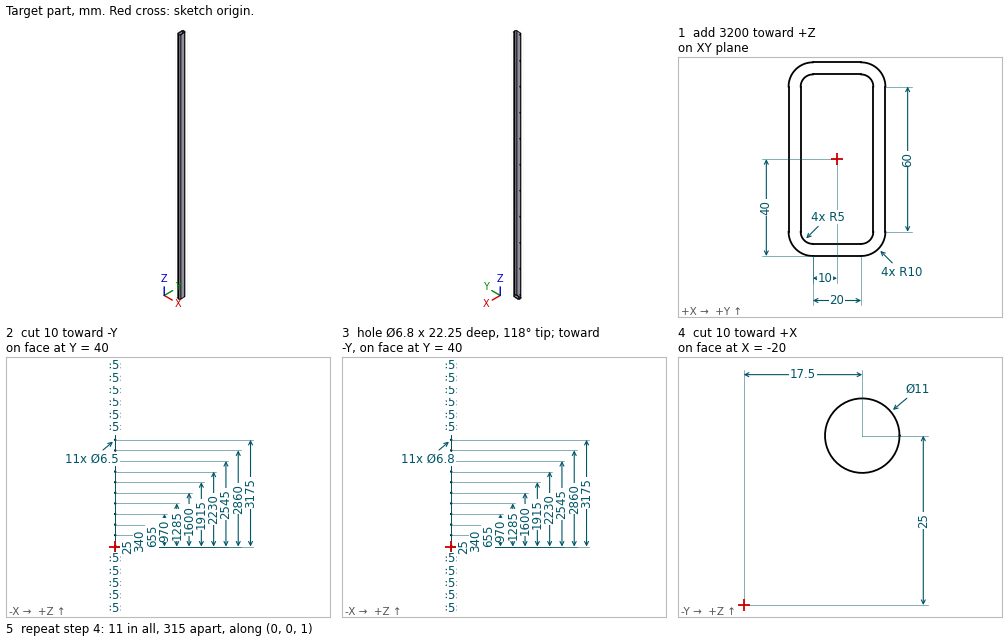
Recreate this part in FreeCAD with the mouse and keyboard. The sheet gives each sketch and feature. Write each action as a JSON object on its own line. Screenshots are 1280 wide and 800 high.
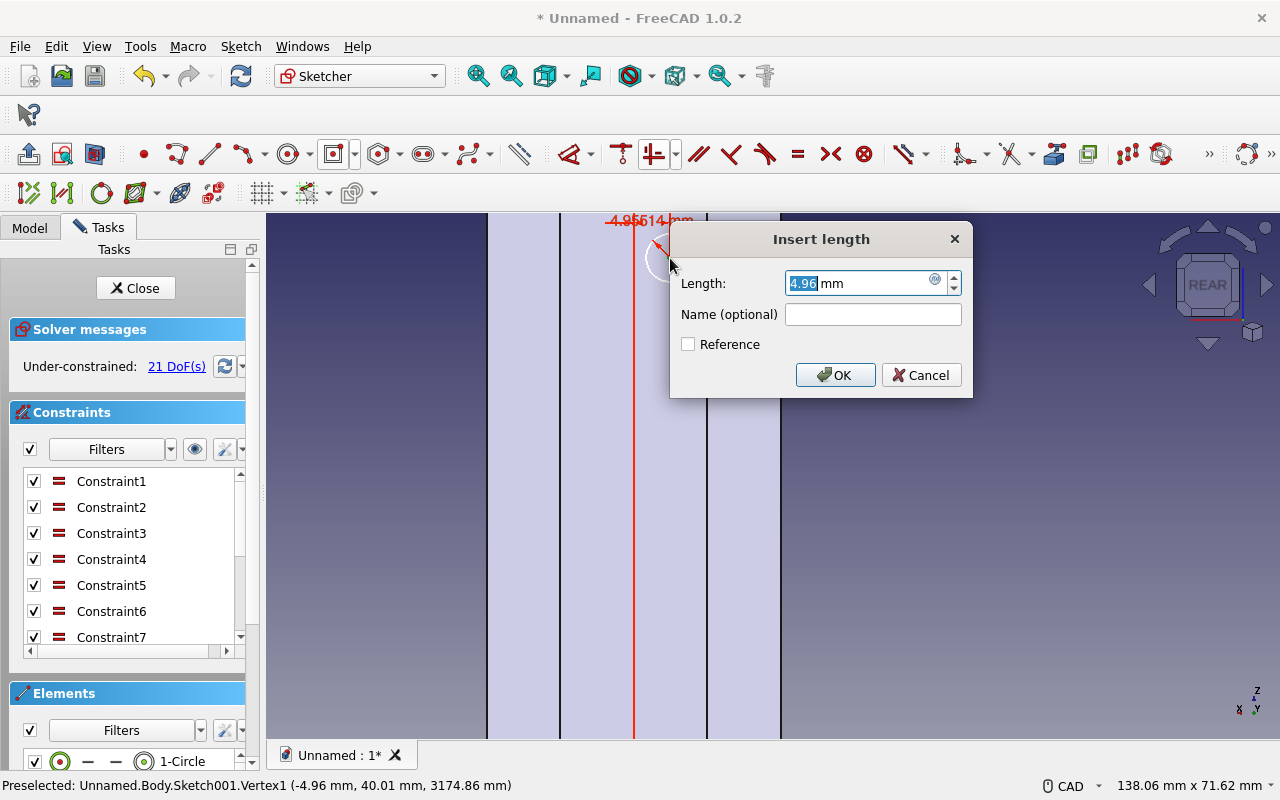
{"action": "type", "text": "5"}
{"action": "key", "text": "Return"}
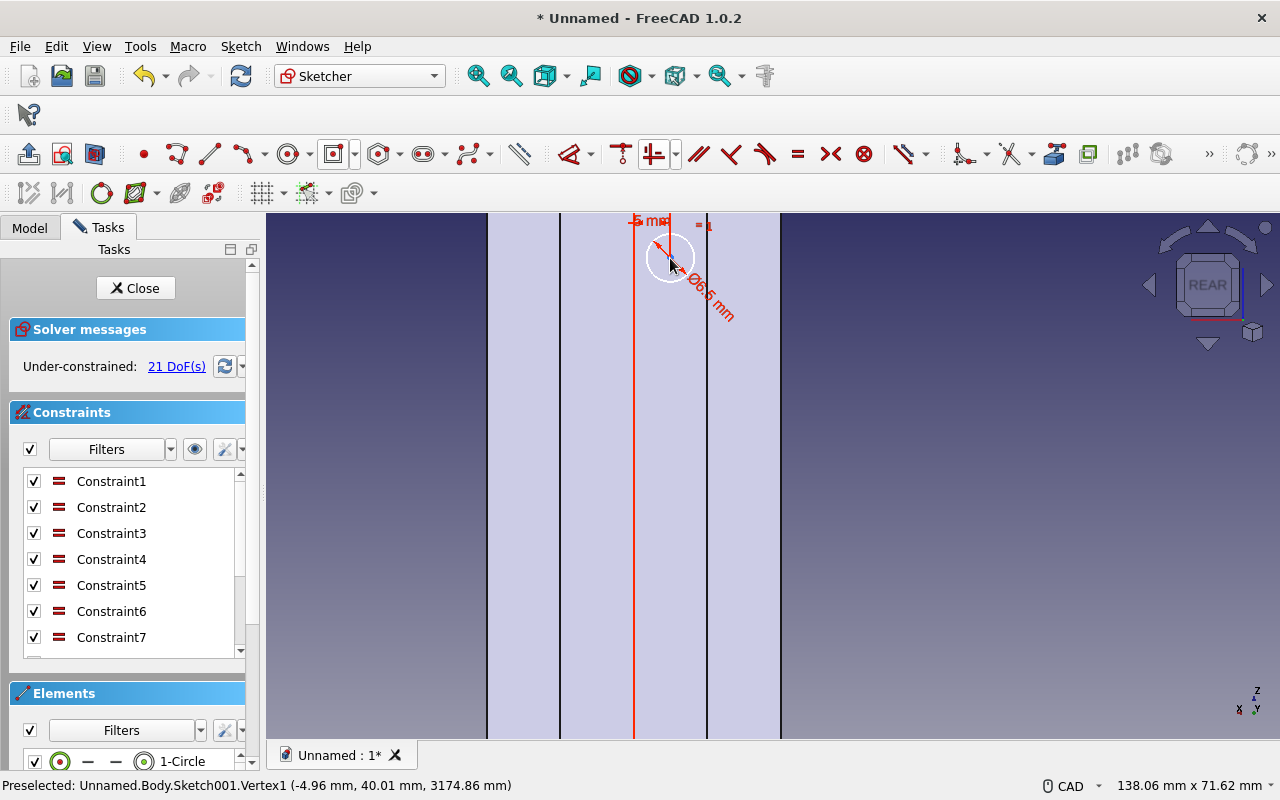
{"action": "scroll", "coordinate": [704, 476], "scroll_direction": "down", "scroll_amount": 15}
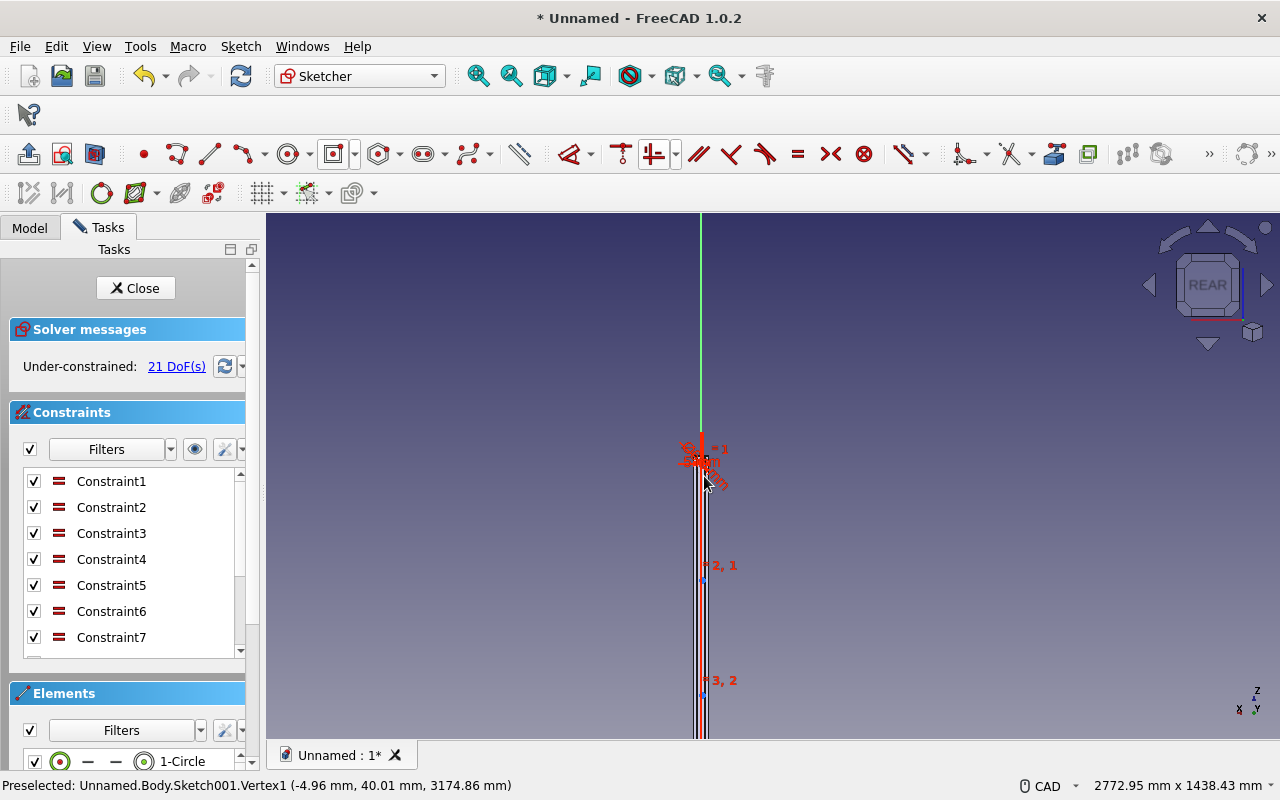
{"action": "scroll", "coordinate": [705, 241], "scroll_direction": "down", "scroll_amount": 6}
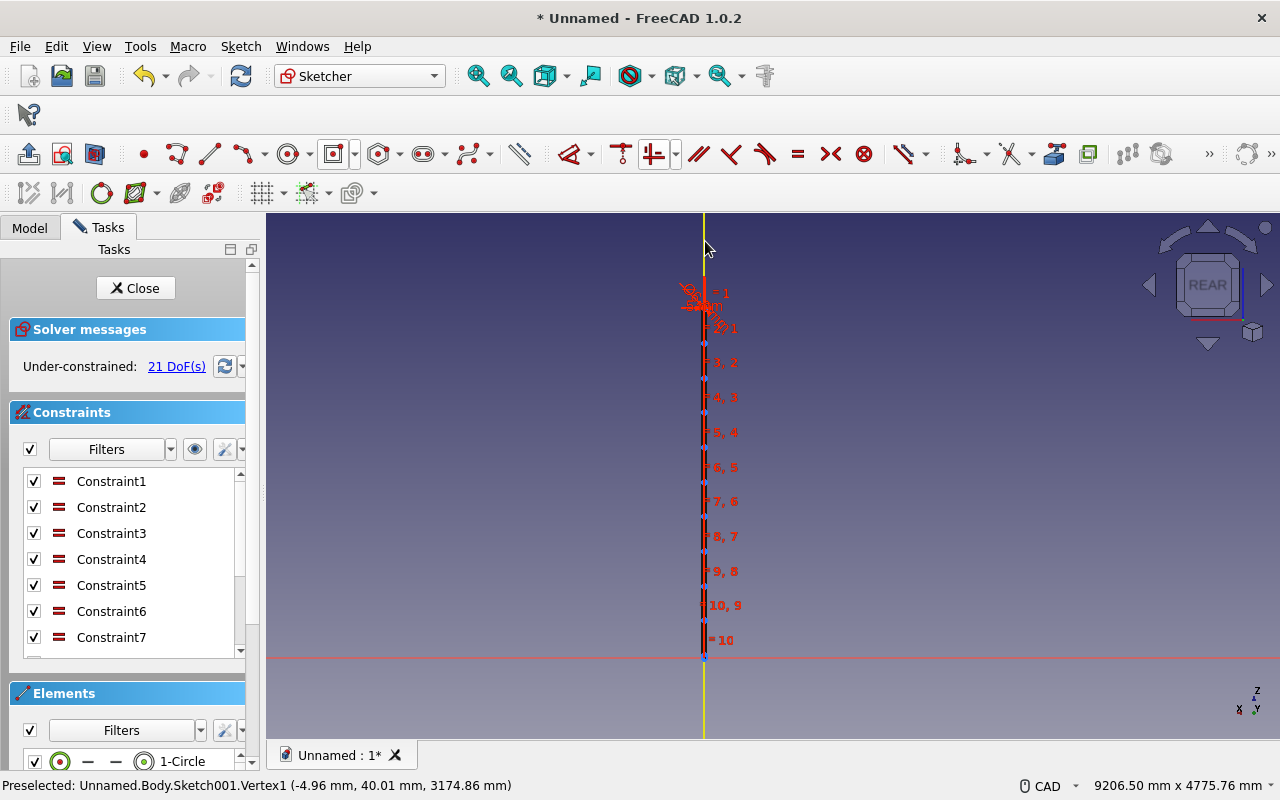
{"action": "scroll", "coordinate": [705, 343], "scroll_direction": "up", "scroll_amount": 22}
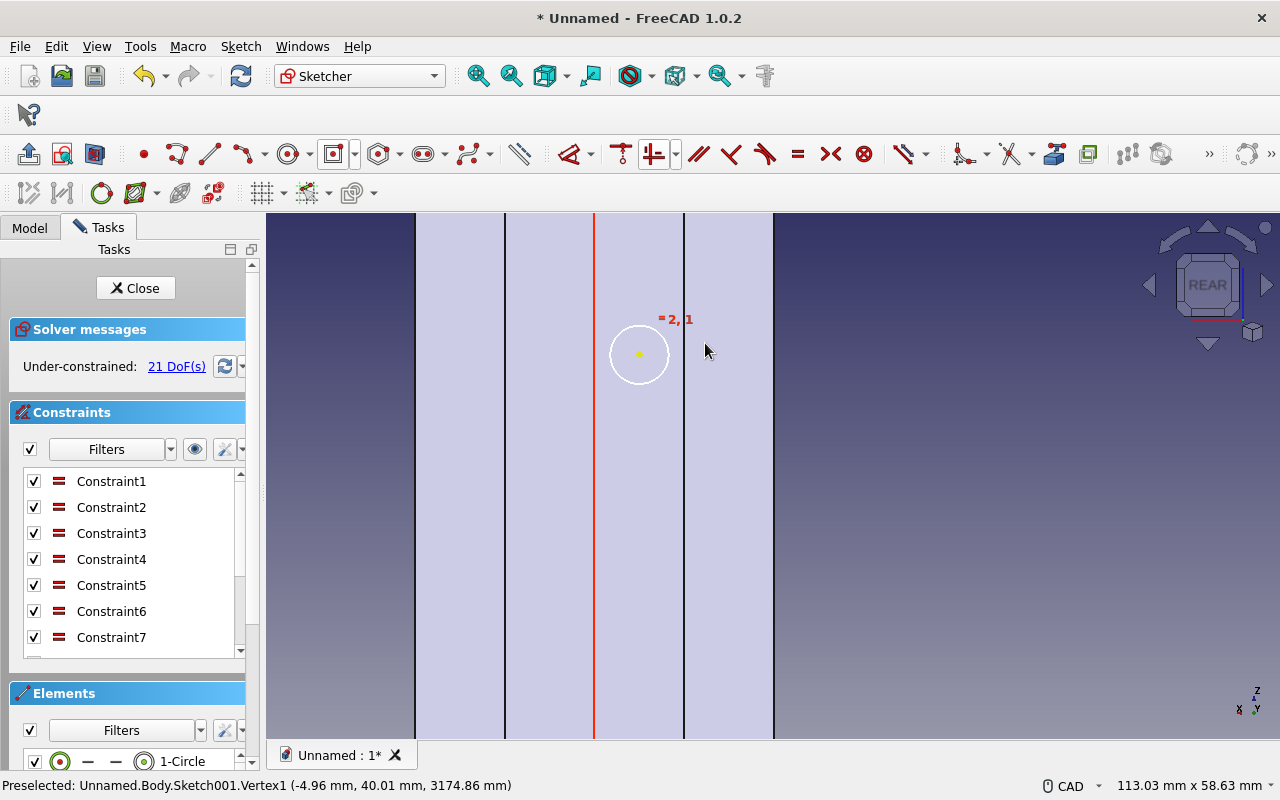
{"action": "left_click", "coordinate": [639, 355]}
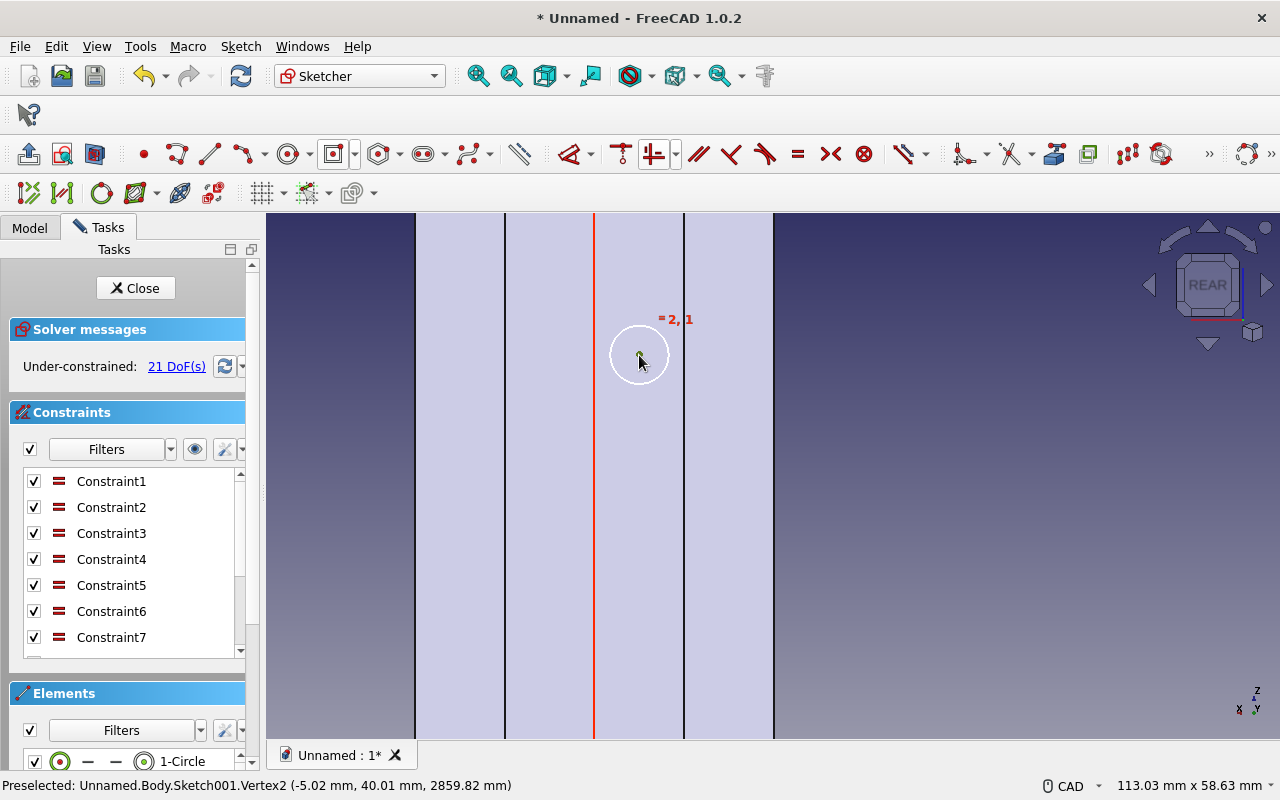
{"action": "key", "text": "l"}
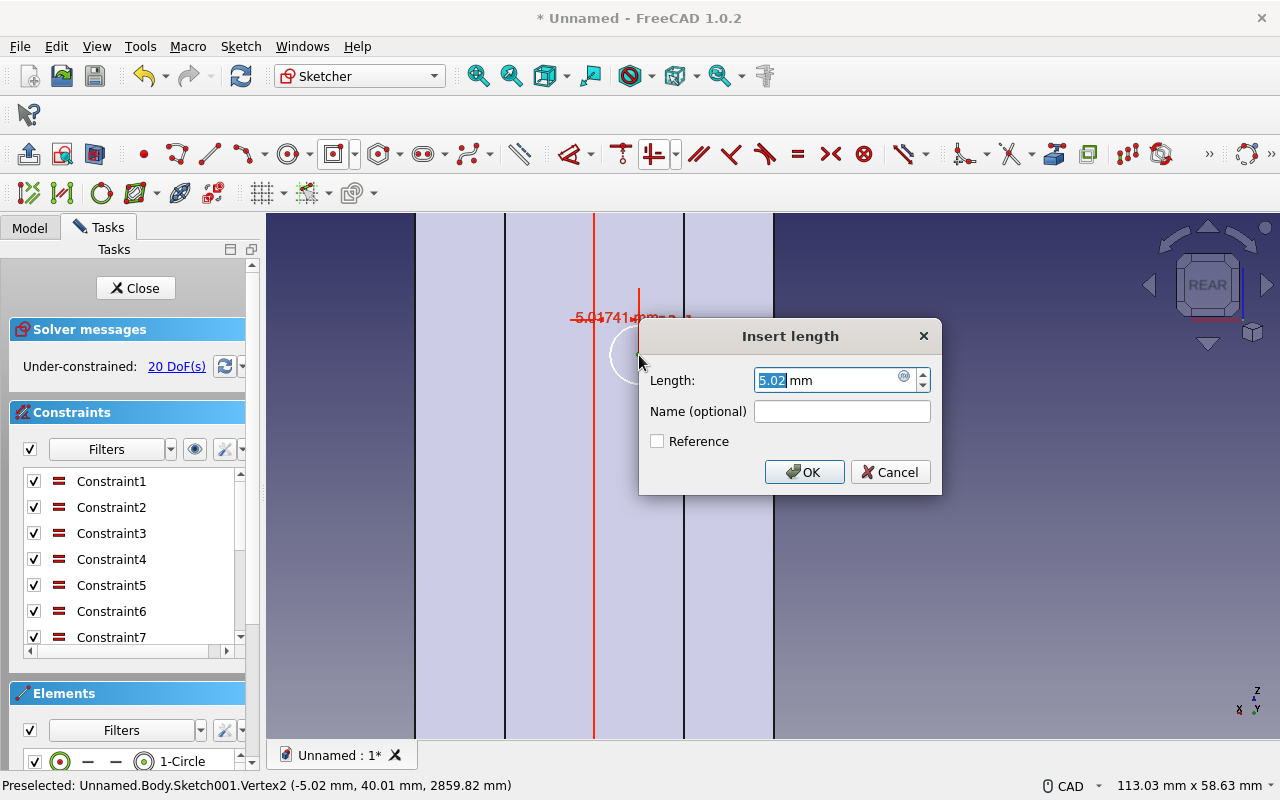
{"action": "type", "text": "5"}
{"action": "key", "text": "Return"}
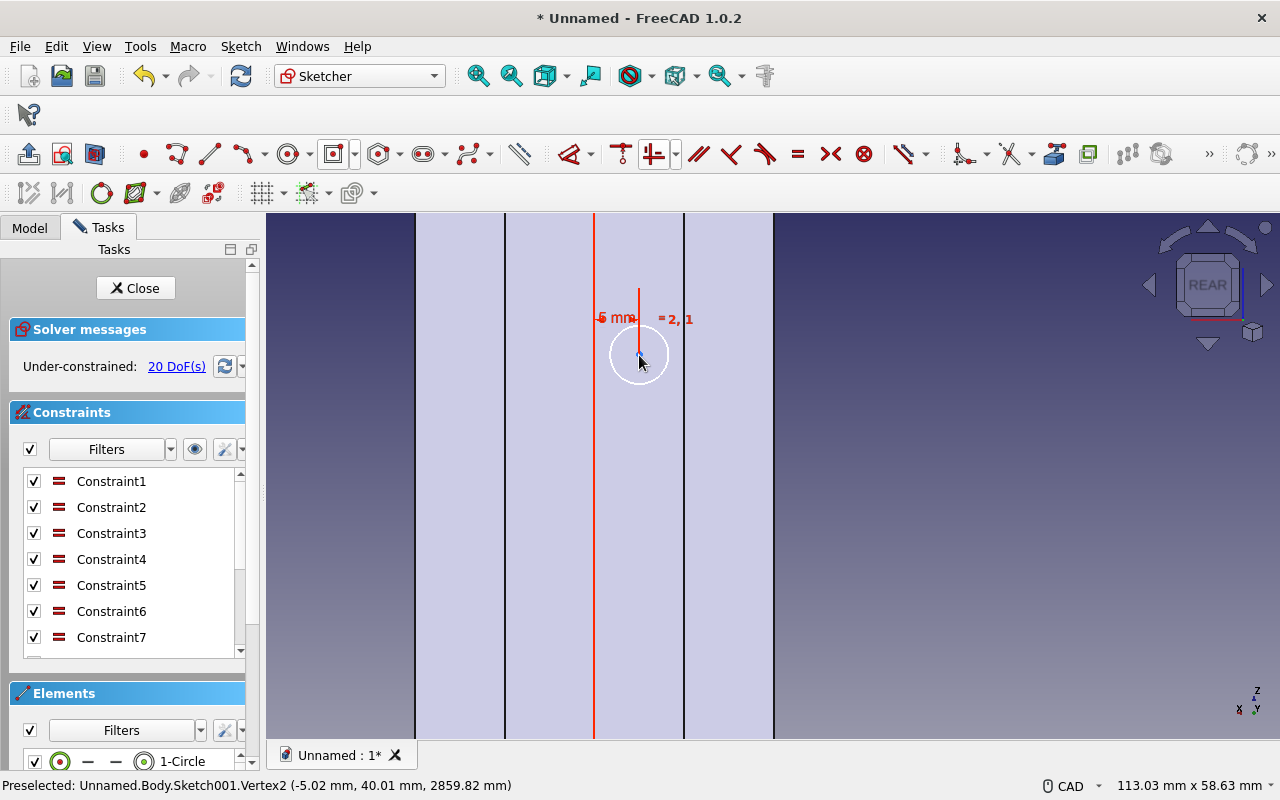
{"action": "scroll", "coordinate": [704, 476], "scroll_direction": "down", "scroll_amount": 15}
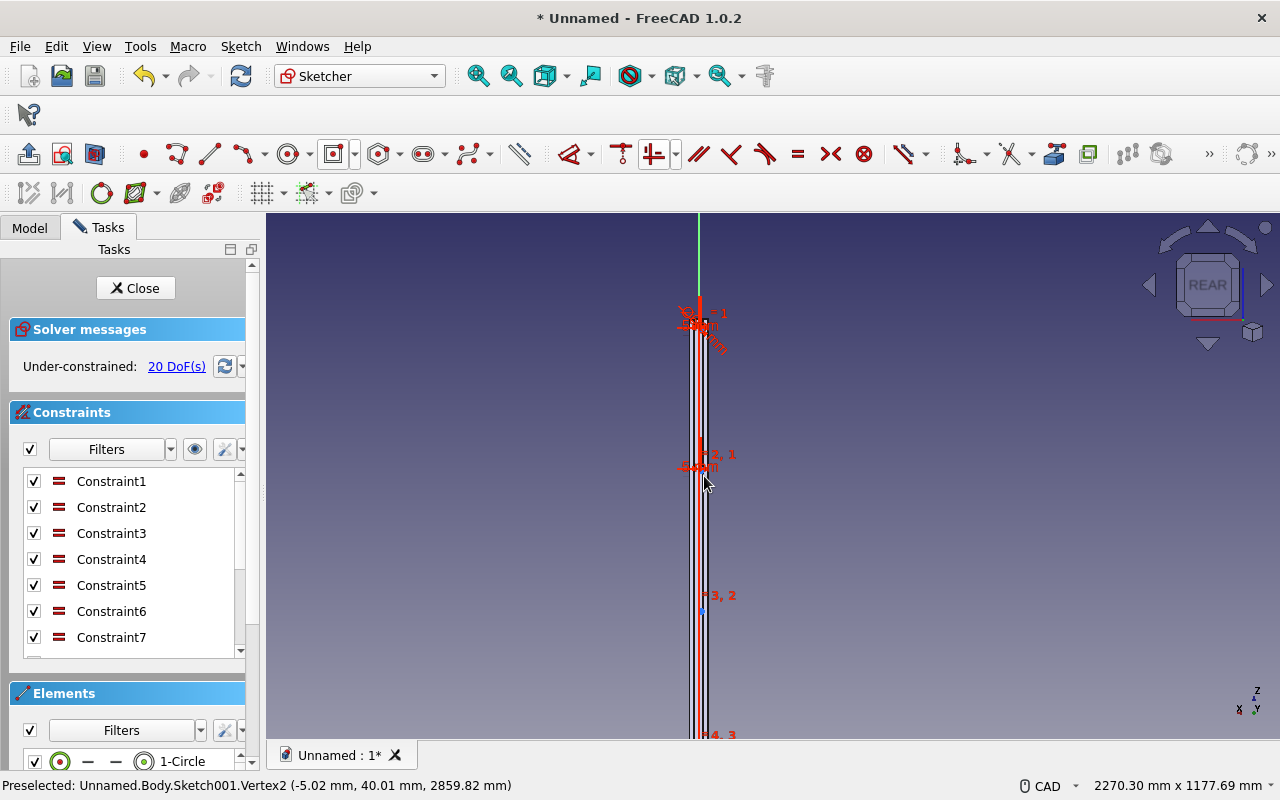
{"action": "scroll", "coordinate": [706, 292], "scroll_direction": "down", "scroll_amount": 7}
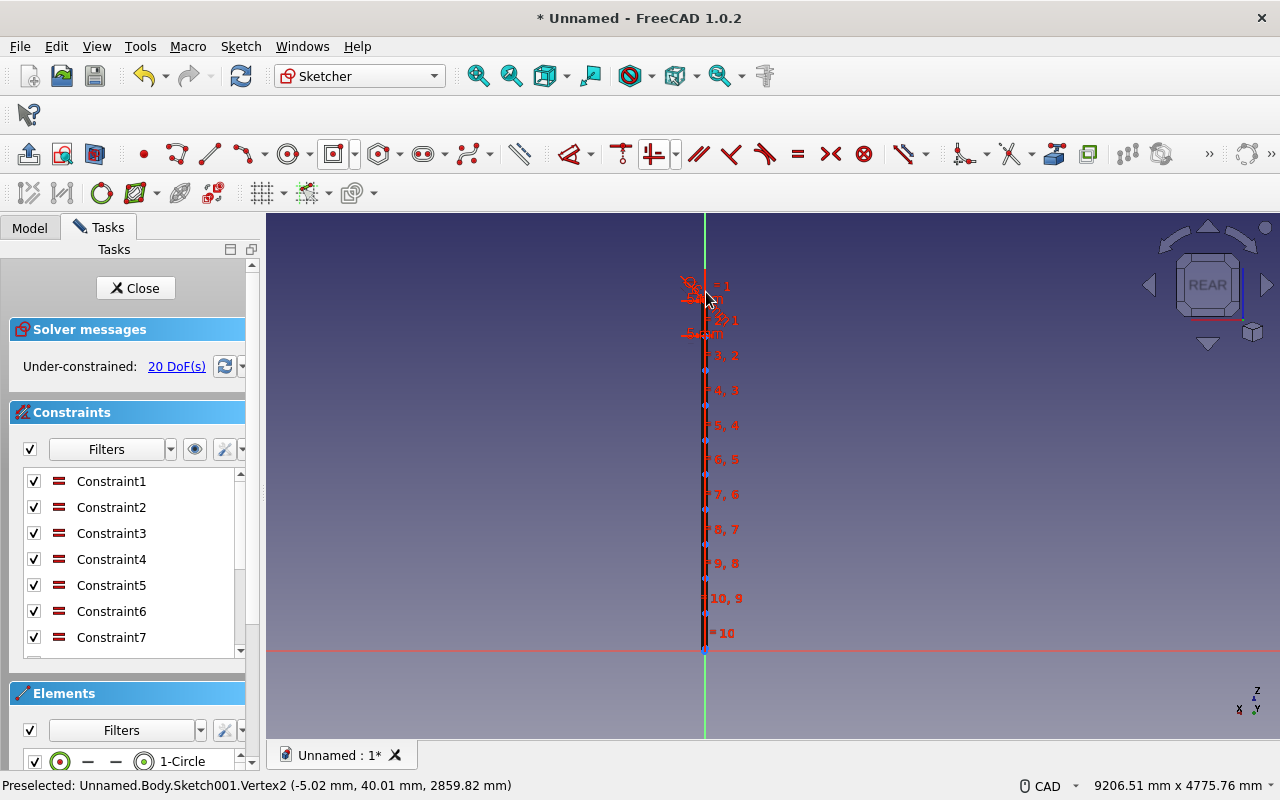
{"action": "scroll", "coordinate": [705, 371], "scroll_direction": "up", "scroll_amount": 22}